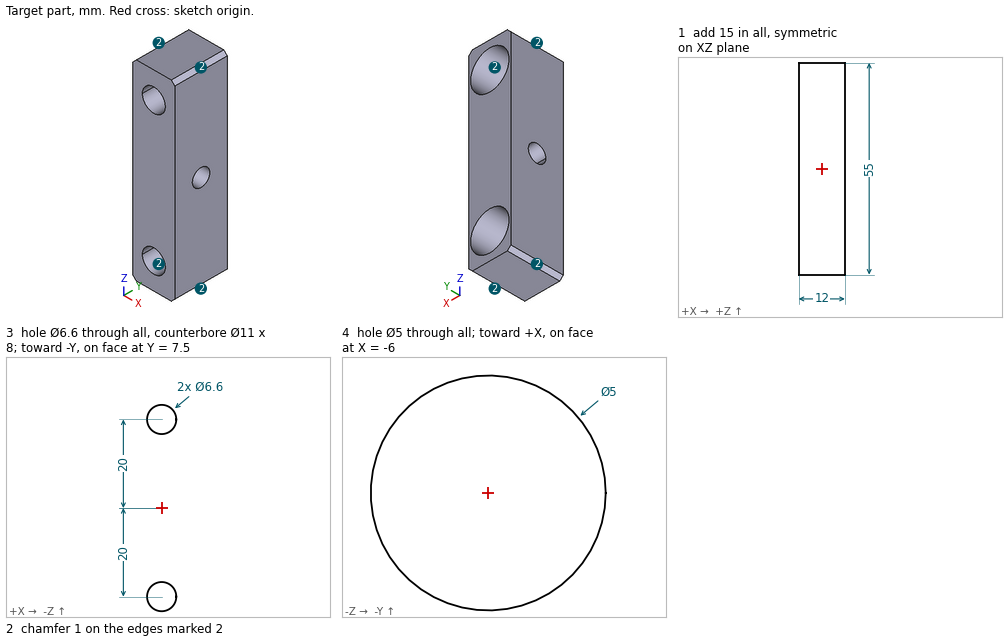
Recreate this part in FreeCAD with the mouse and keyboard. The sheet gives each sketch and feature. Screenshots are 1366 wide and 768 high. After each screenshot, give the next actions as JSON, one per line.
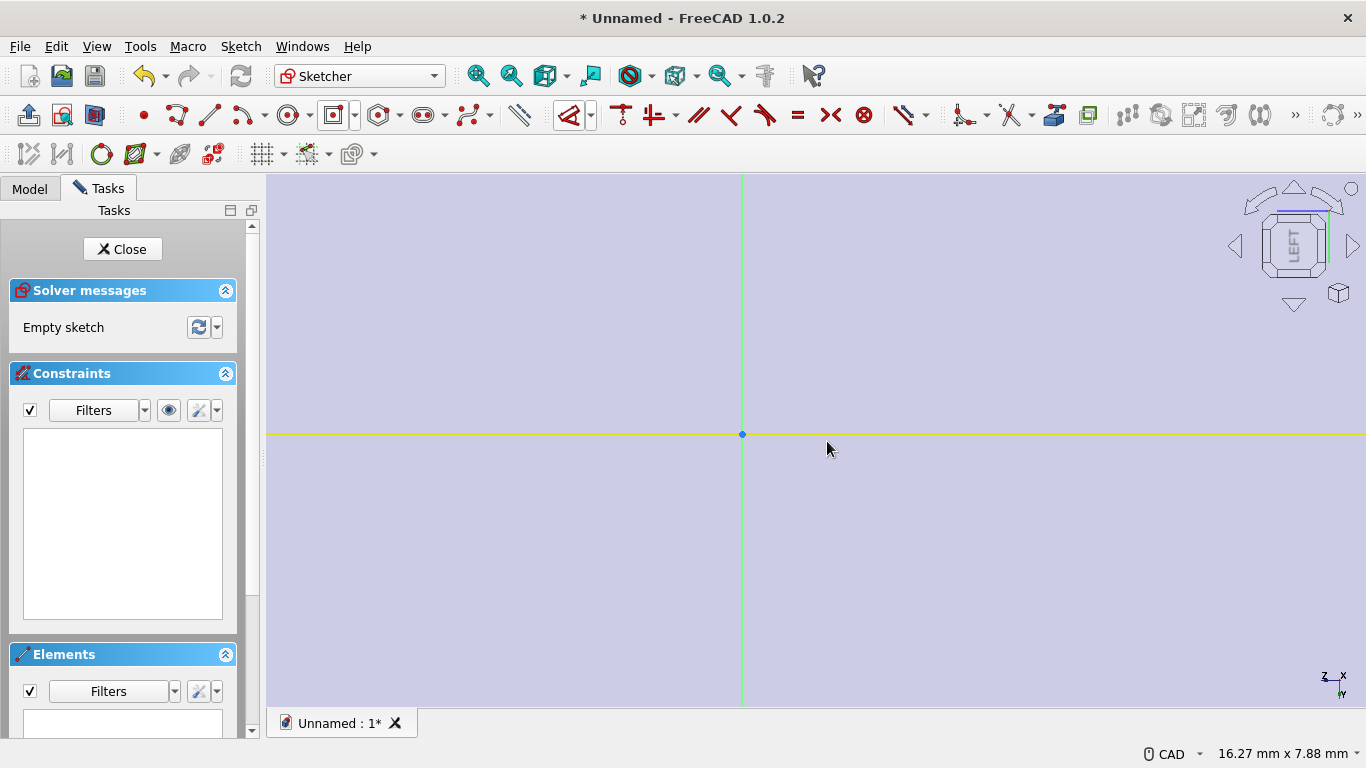
{"action": "left_click", "coordinate": [288, 116]}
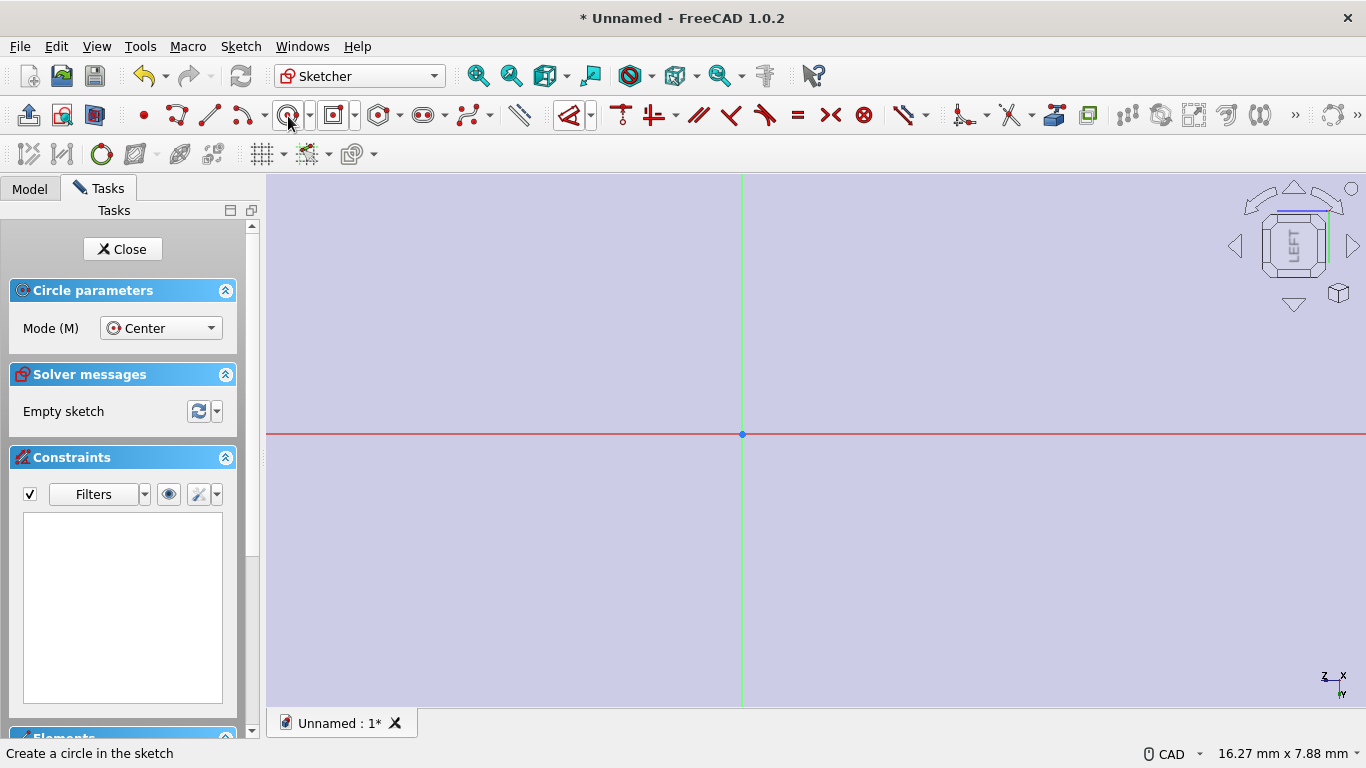
{"action": "left_click", "coordinate": [742, 434]}
{"action": "mouse_move", "coordinate": [862, 315]}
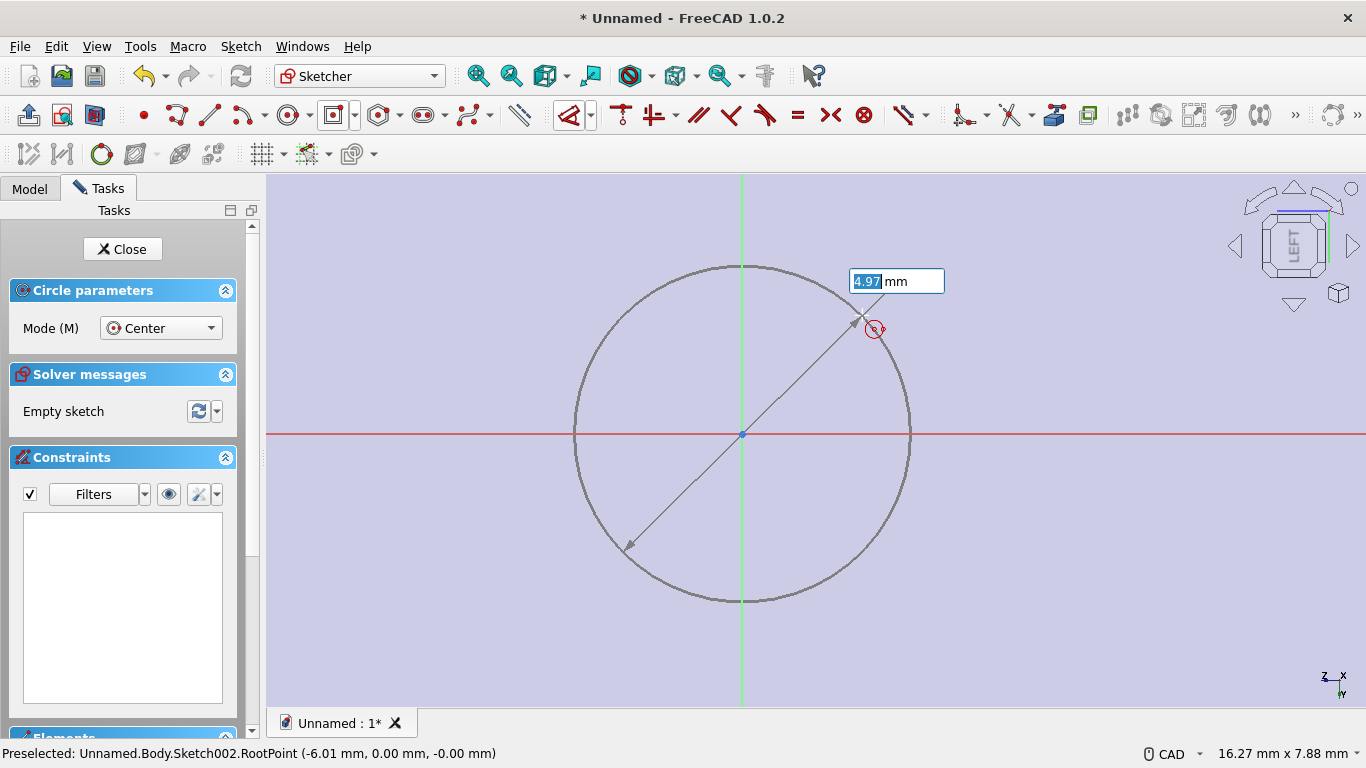
{"action": "type", "text": "5"}
{"action": "key", "text": "Return"}
{"action": "key", "text": "Escape"}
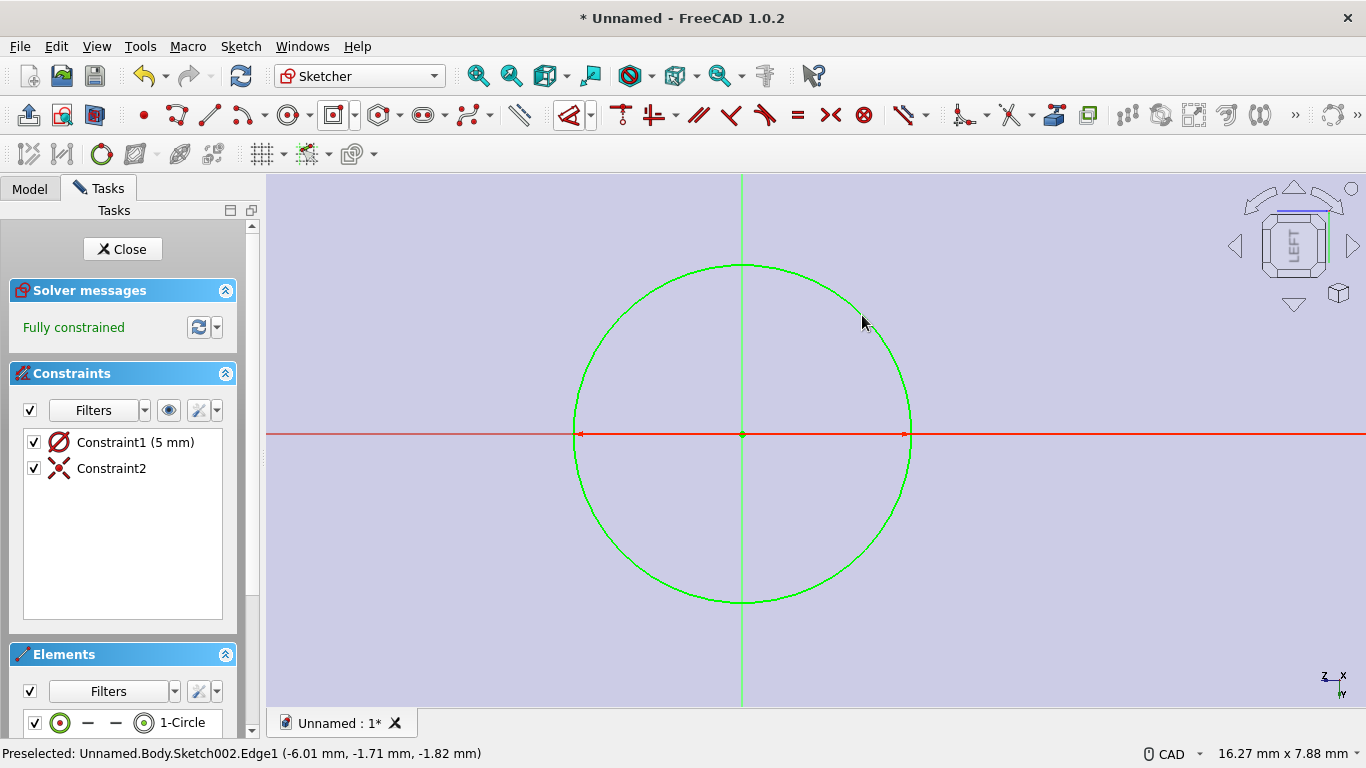
{"action": "left_click", "coordinate": [123, 249]}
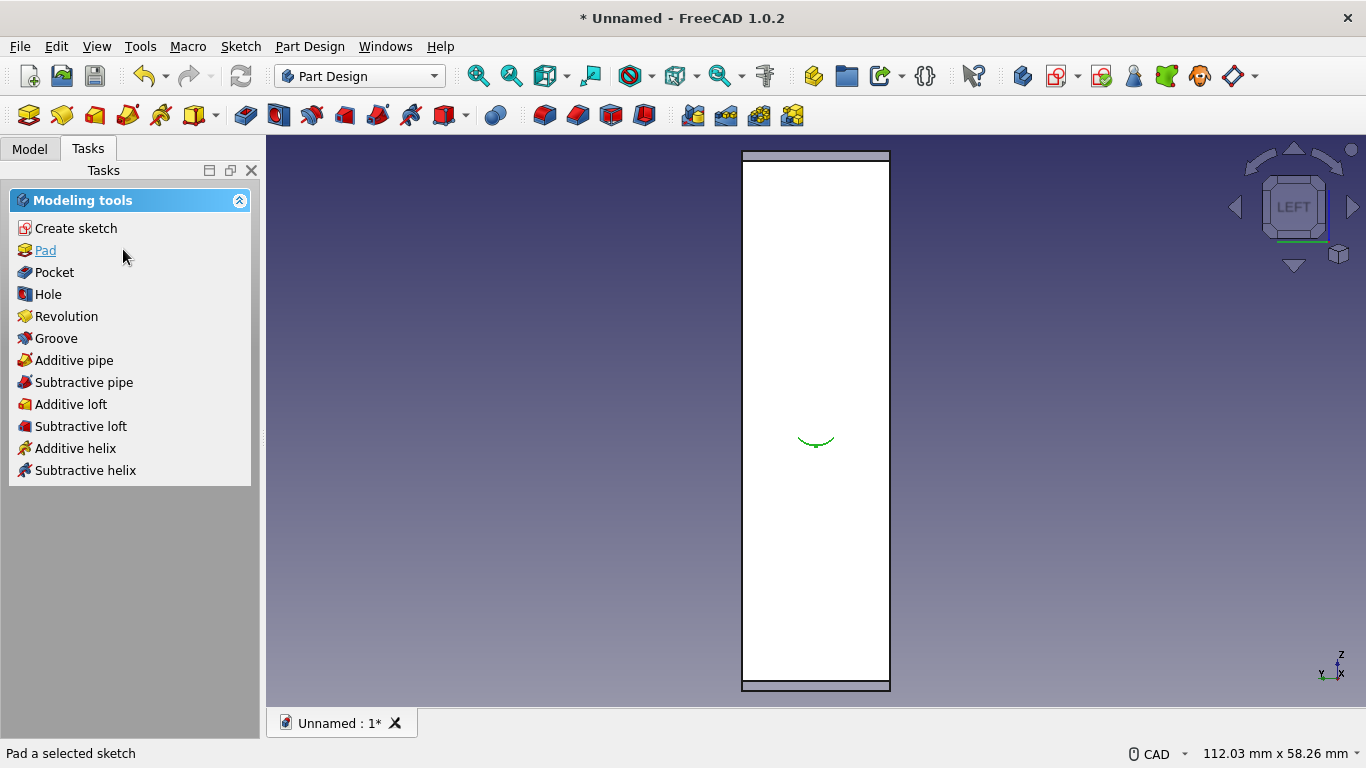
{"action": "left_click", "coordinate": [279, 116]}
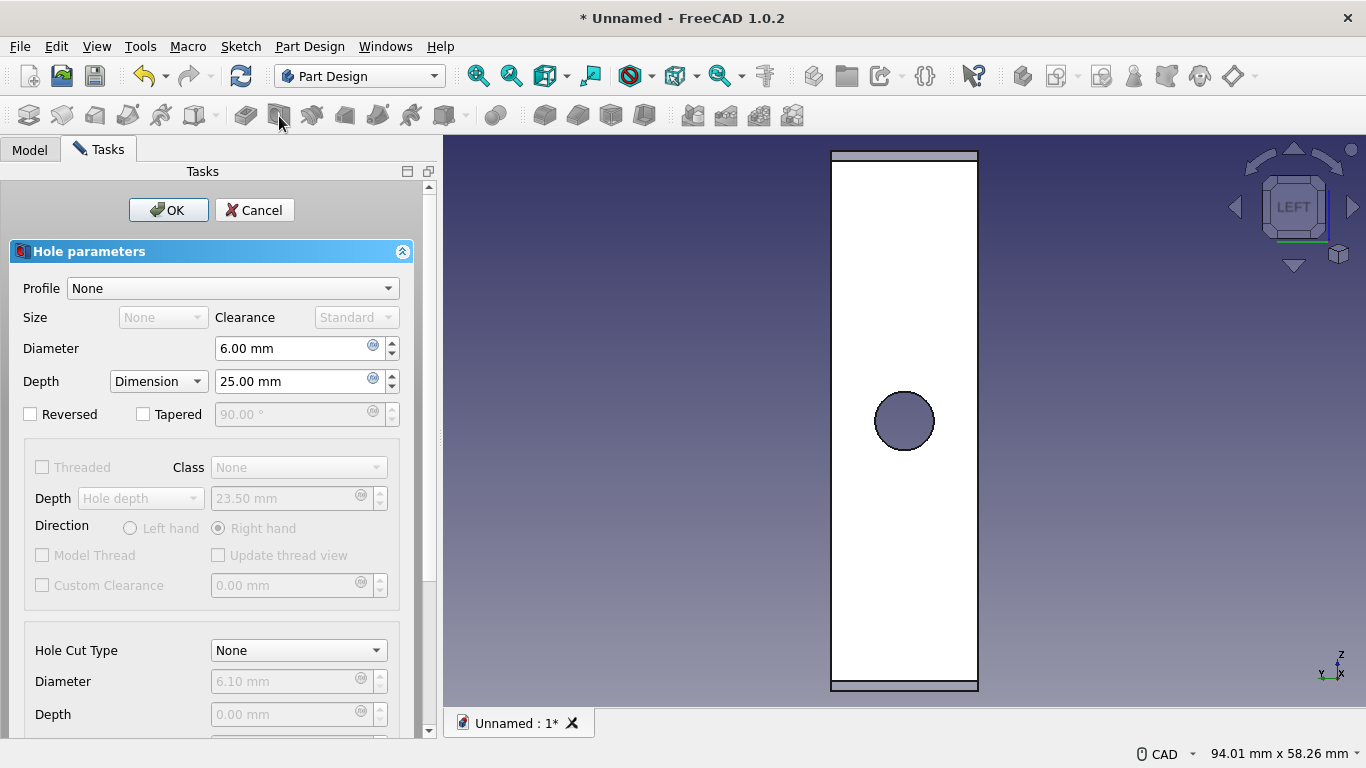
{"action": "triple_click", "coordinate": [300, 348]}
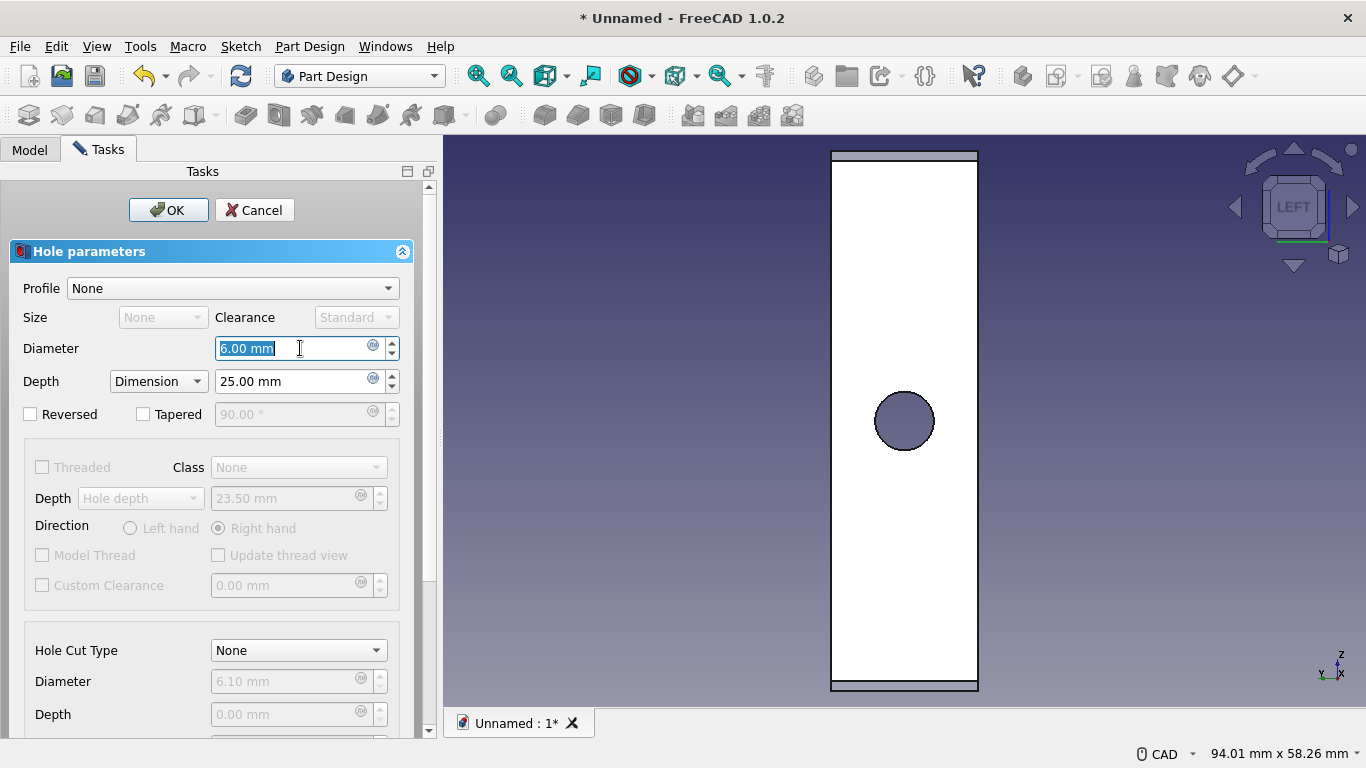
{"action": "type", "text": "5"}
{"action": "key", "text": "Tab"}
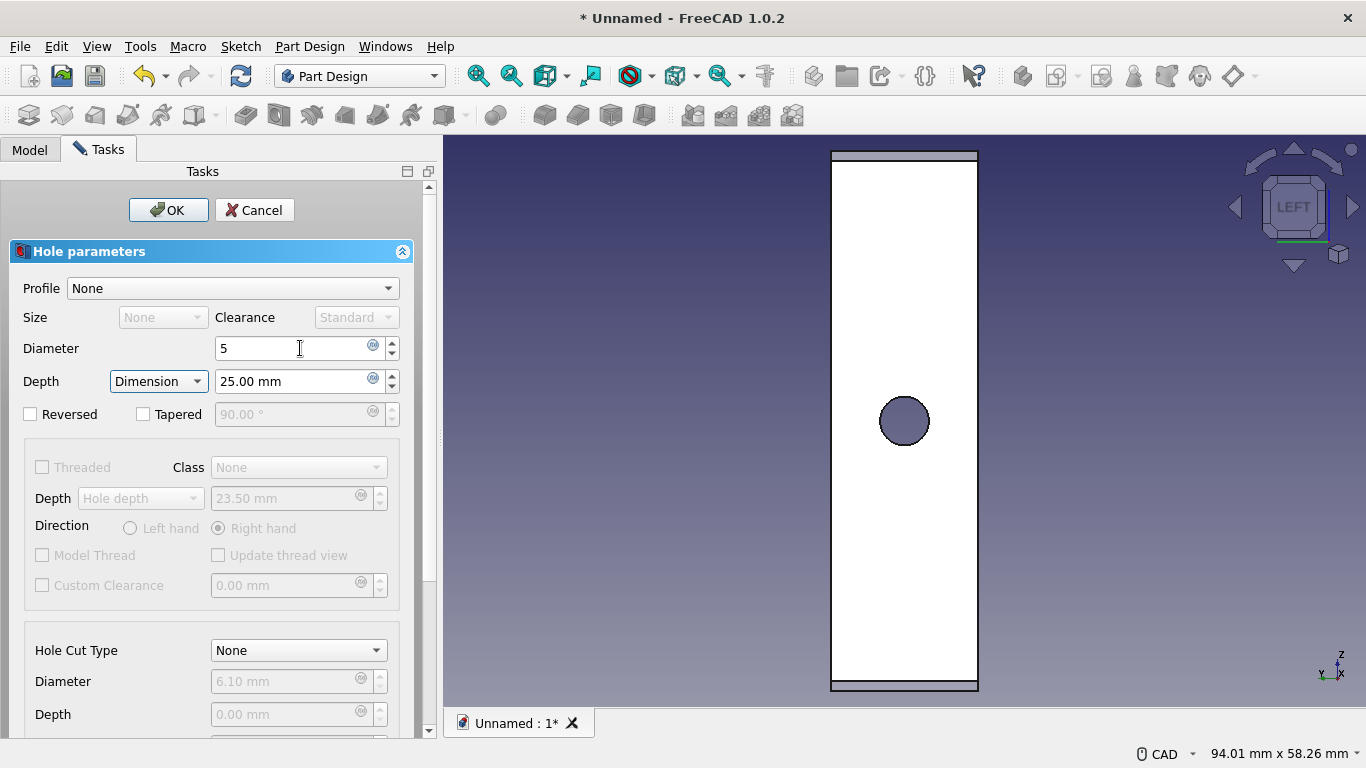
{"action": "left_click", "coordinate": [160, 382]}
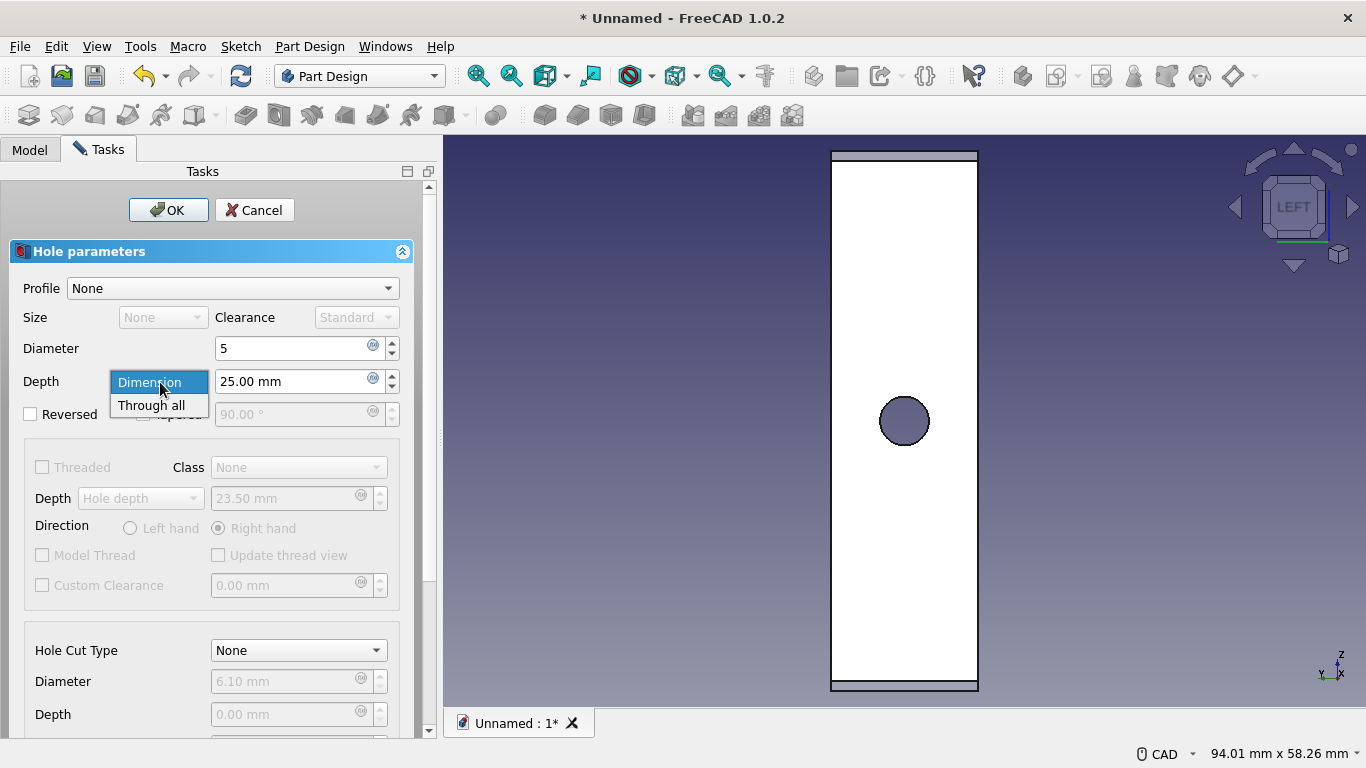
{"action": "left_click", "coordinate": [158, 406]}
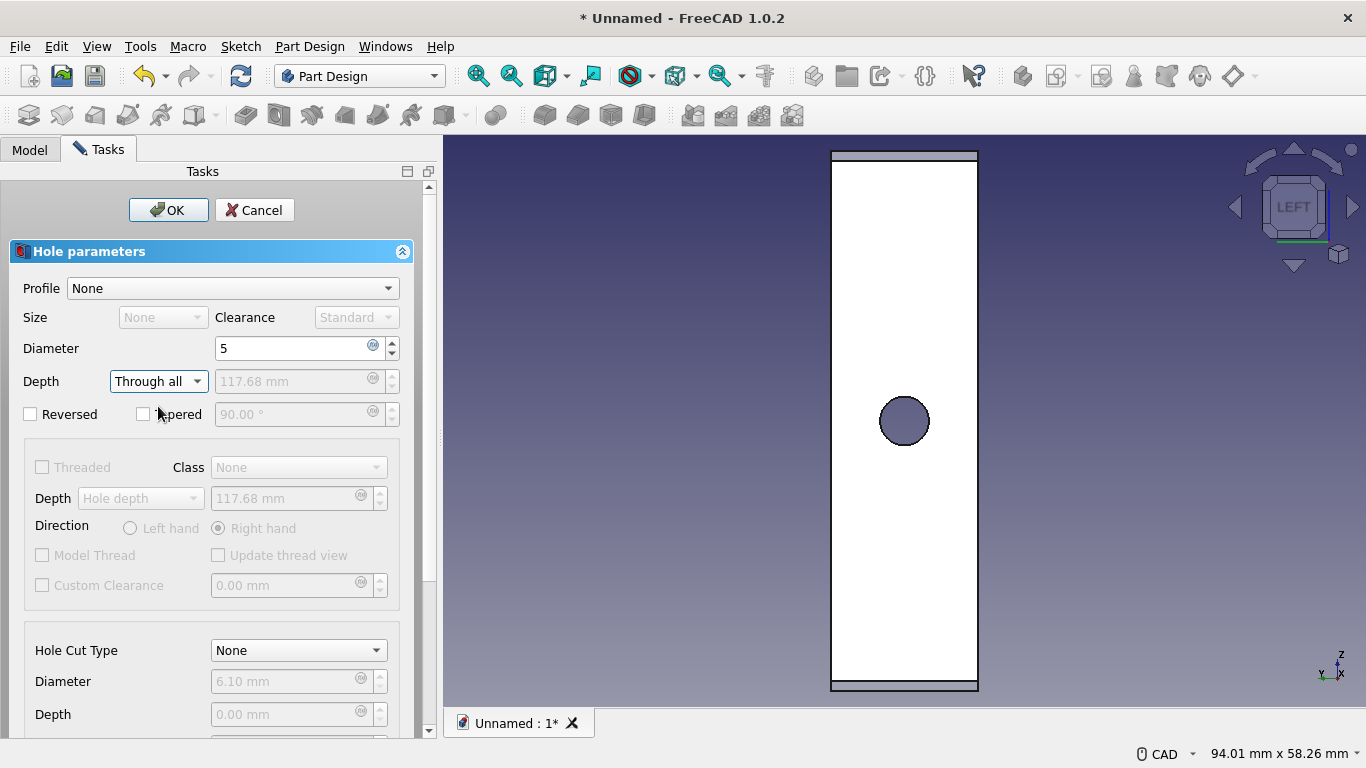
{"action": "left_click", "coordinate": [169, 210]}